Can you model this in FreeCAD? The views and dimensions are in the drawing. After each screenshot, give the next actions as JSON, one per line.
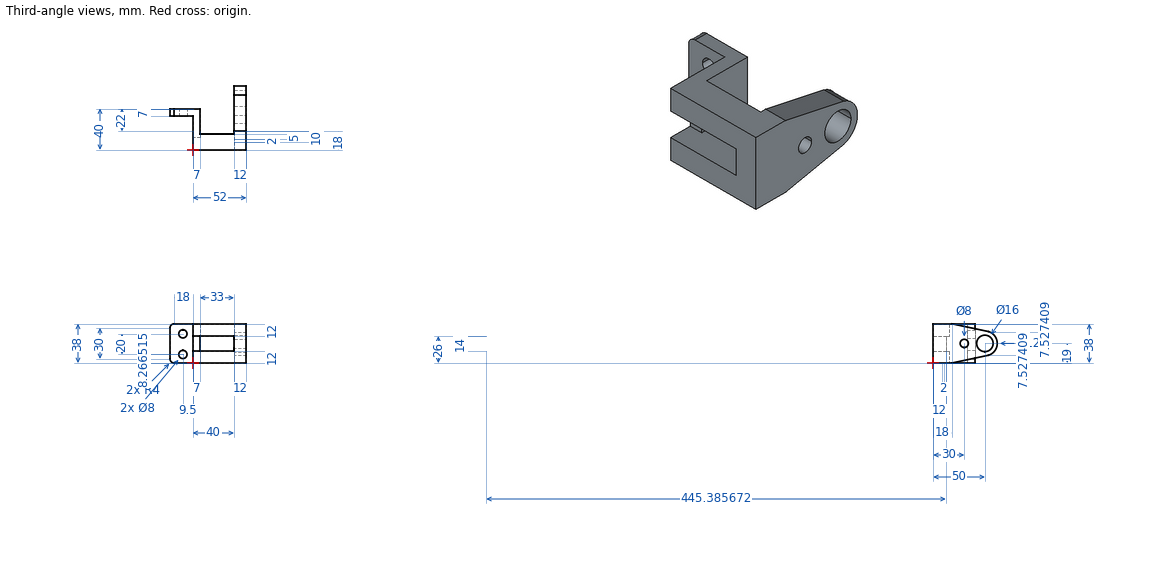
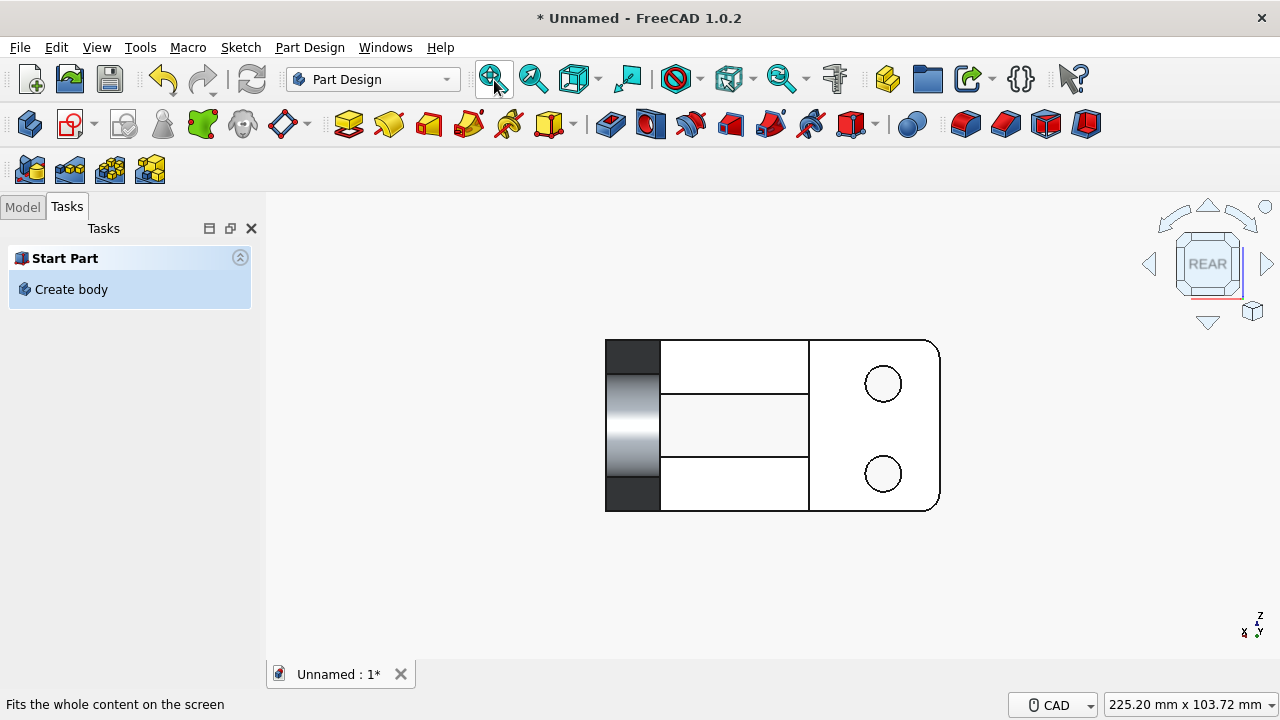
{"action": "left_click", "coordinate": [692, 366]}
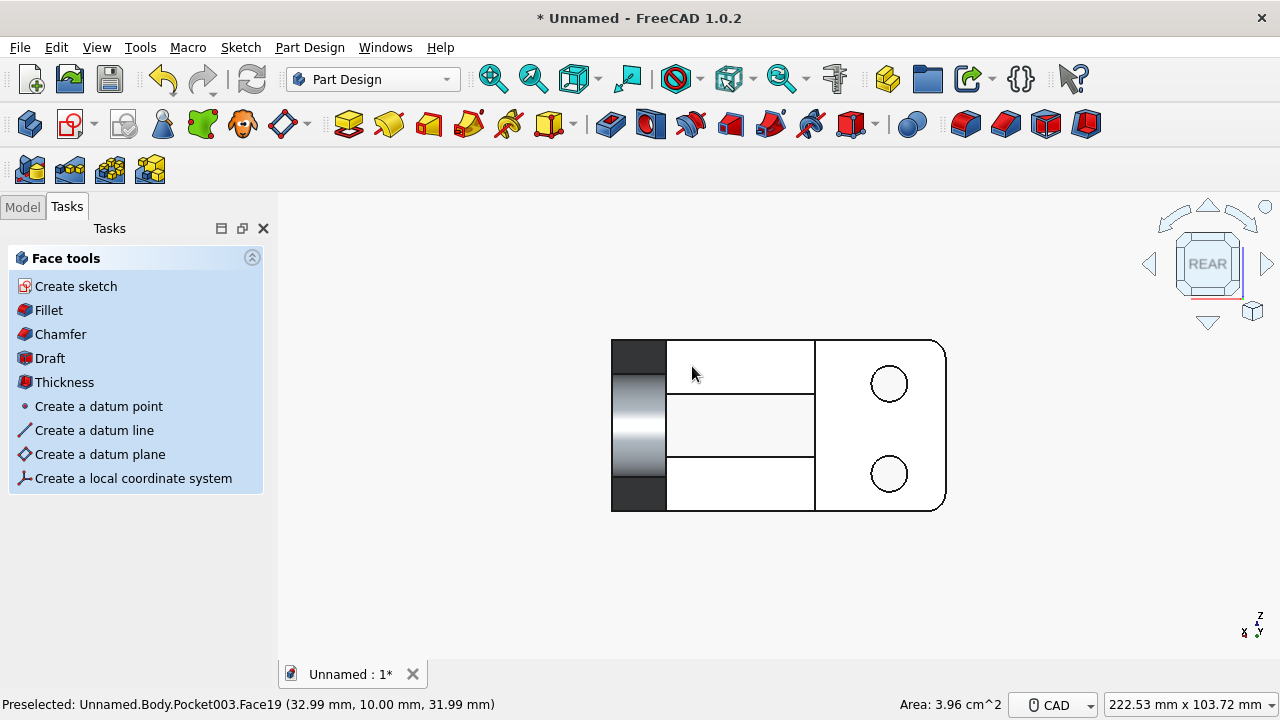
{"action": "left_click", "coordinate": [70, 124]}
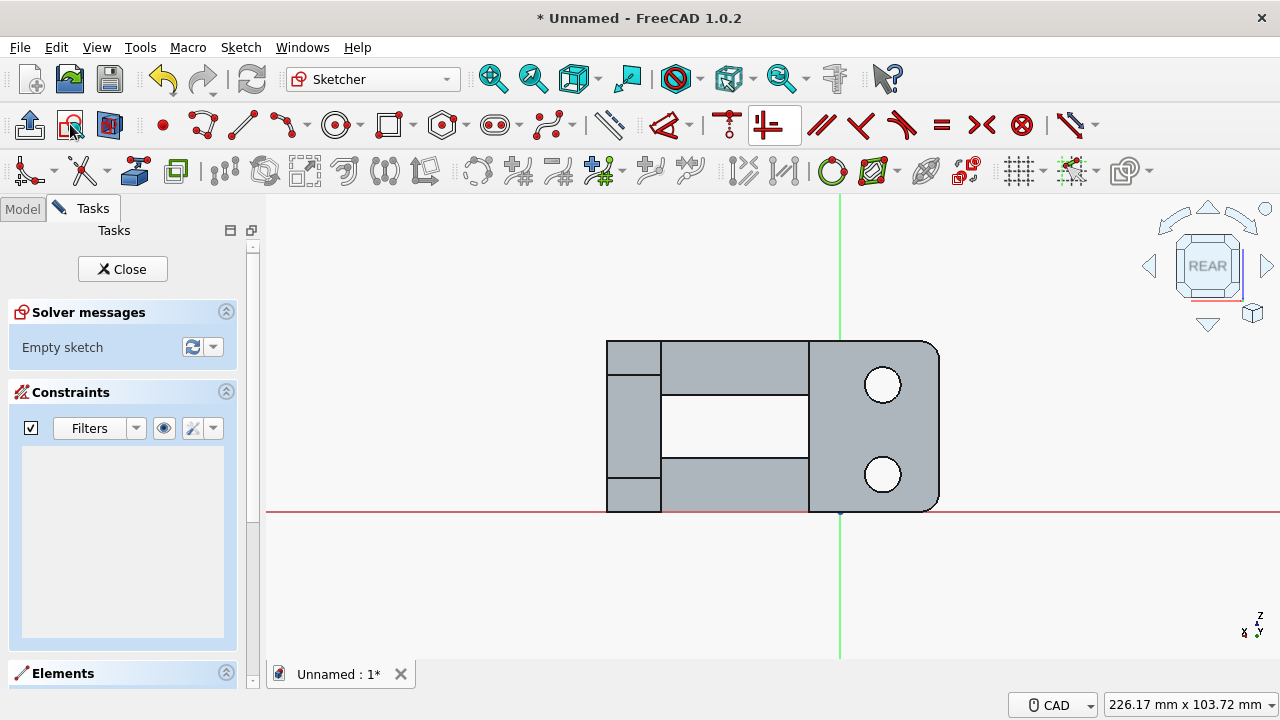
{"action": "scroll", "coordinate": [807, 427], "scroll_direction": "up", "scroll_amount": 3}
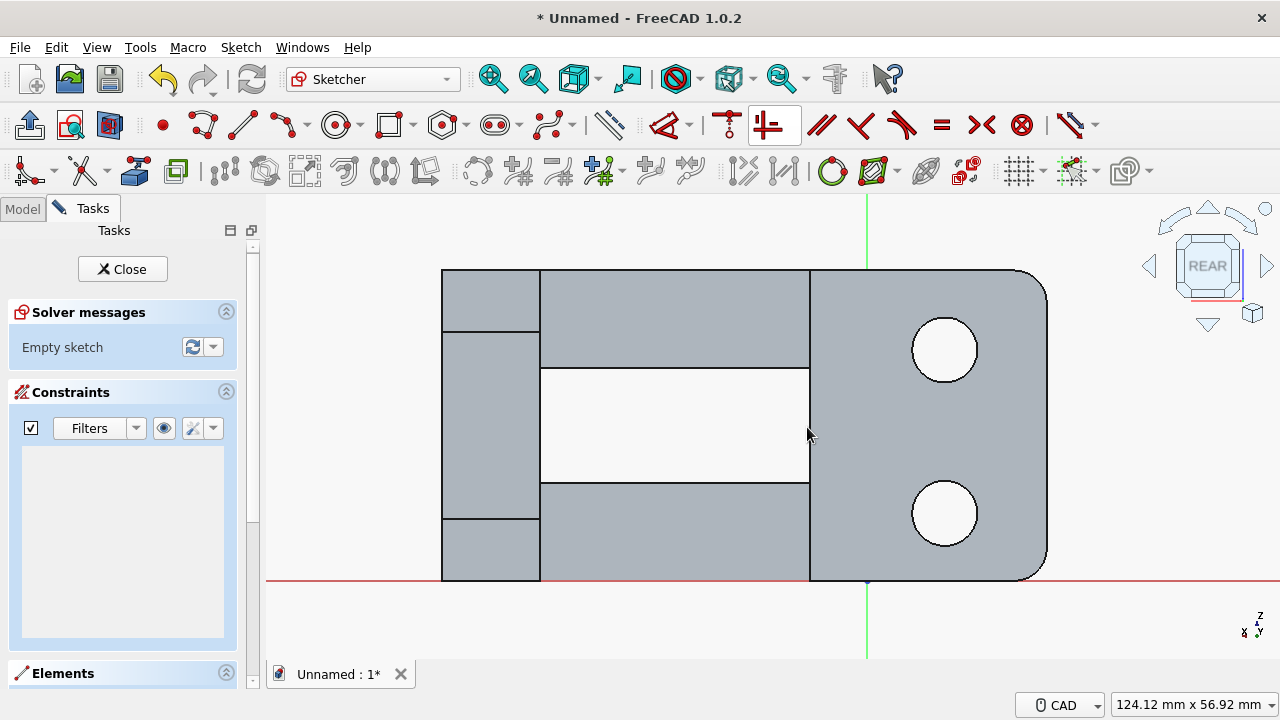
{"action": "left_click", "coordinate": [390, 126]}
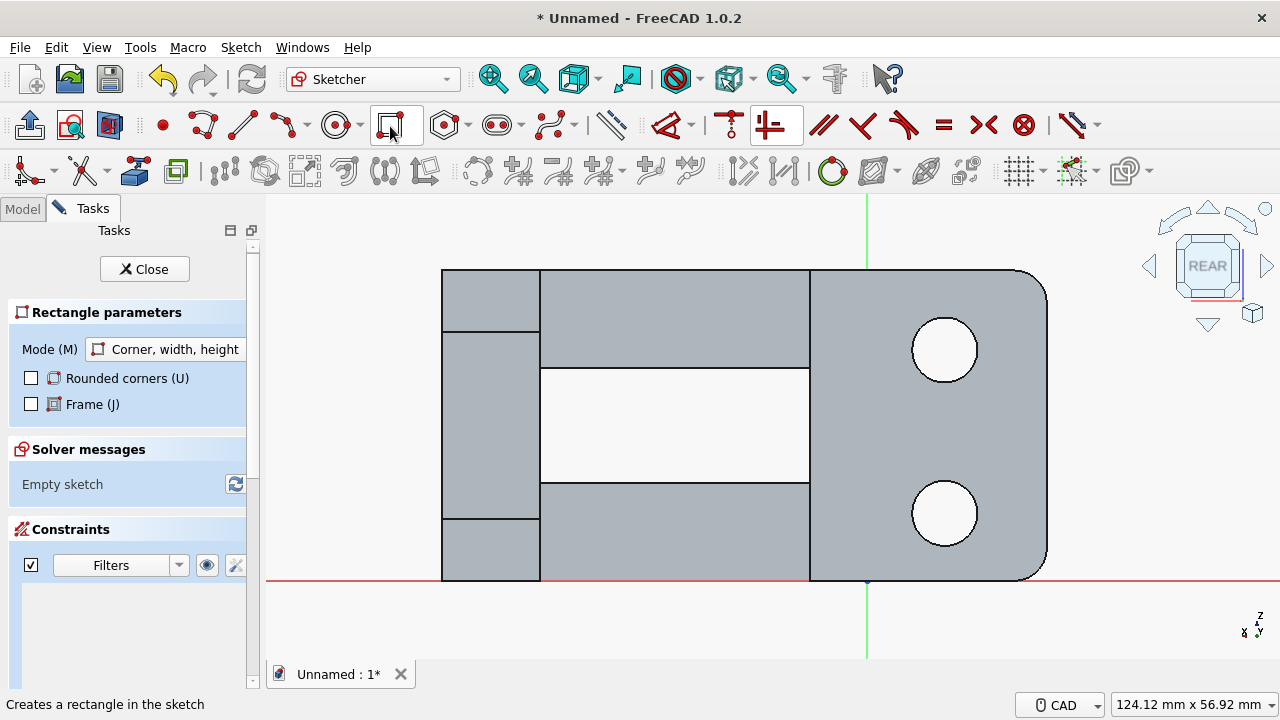
{"action": "left_click", "coordinate": [540, 270]}
{"action": "left_click", "coordinate": [810, 368]}
{"action": "key", "text": "Escape"}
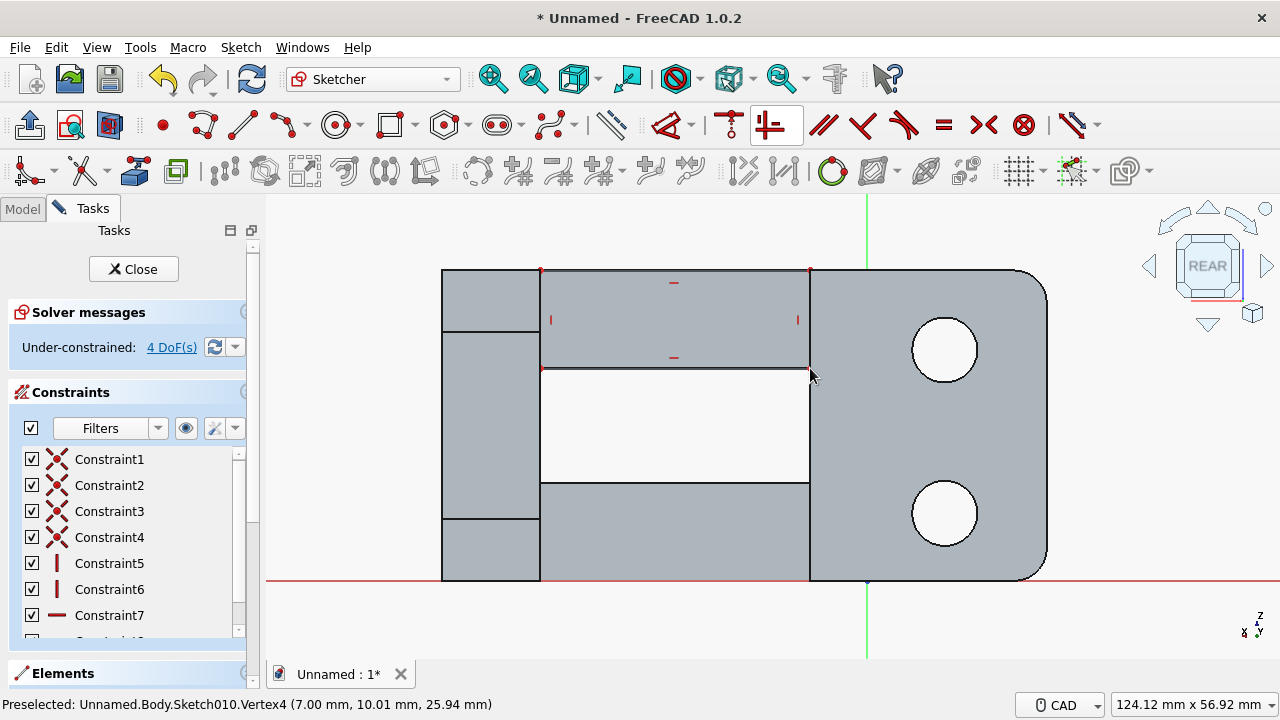
{"action": "left_click", "coordinate": [666, 126]}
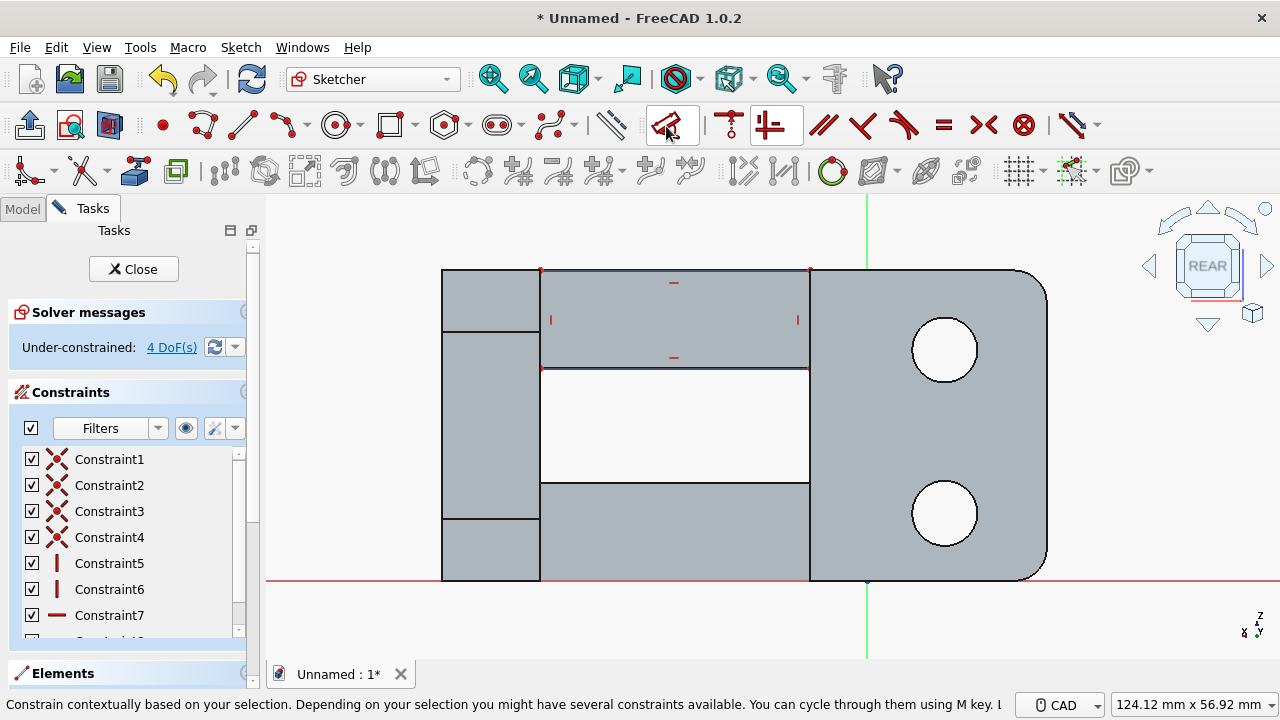
{"action": "left_click", "coordinate": [540, 300]}
{"action": "left_click", "coordinate": [506, 320]}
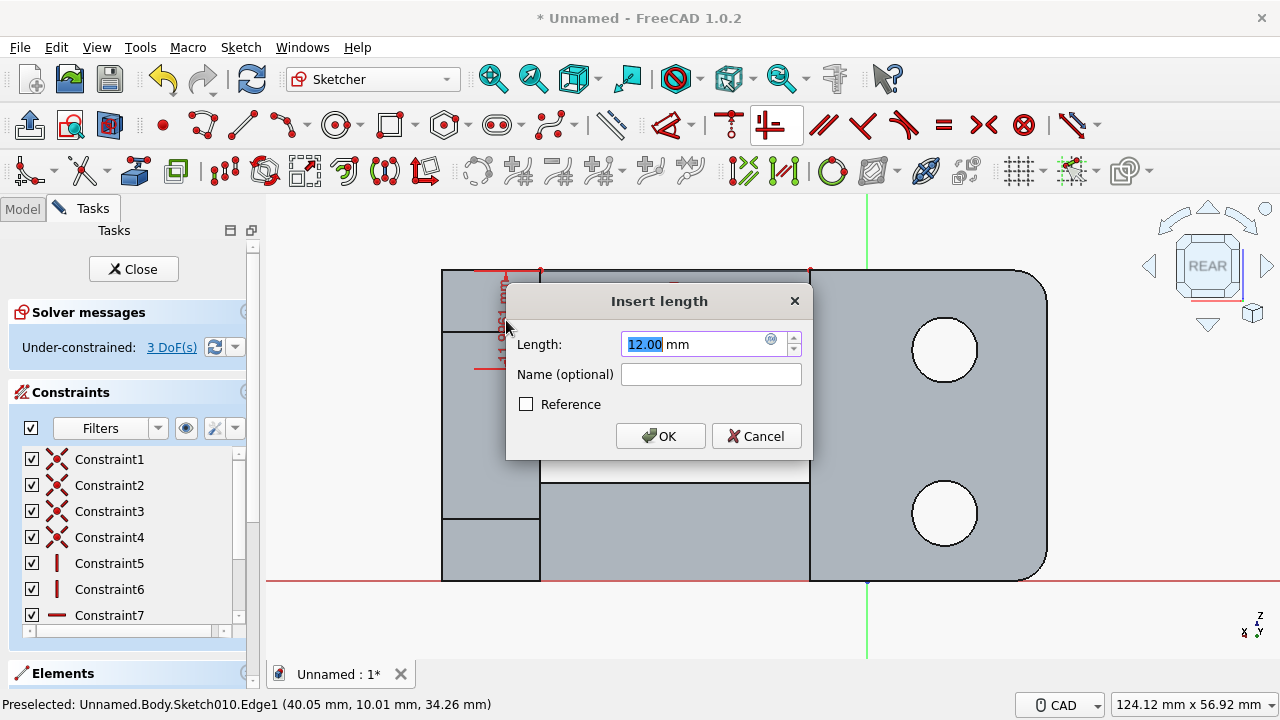
{"action": "type", "text": "12"}
{"action": "key", "text": "Return"}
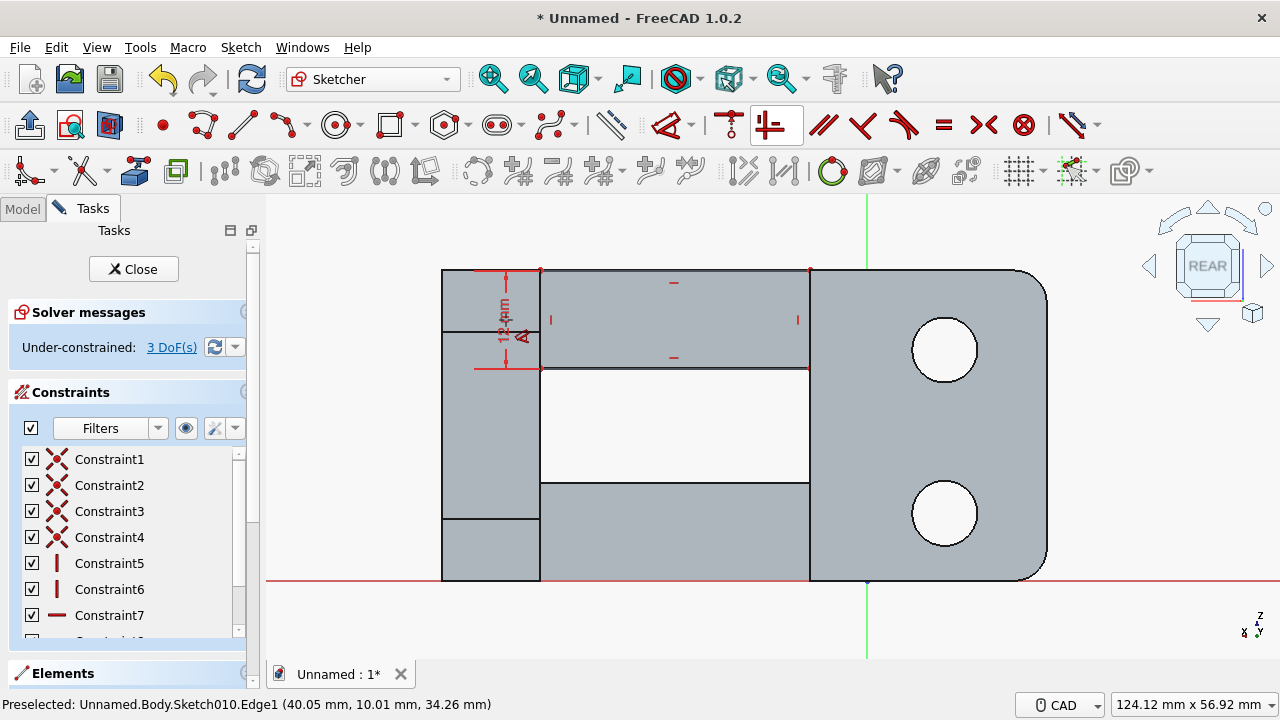
{"action": "left_click", "coordinate": [621, 369]}
{"action": "left_click", "coordinate": [675, 335]}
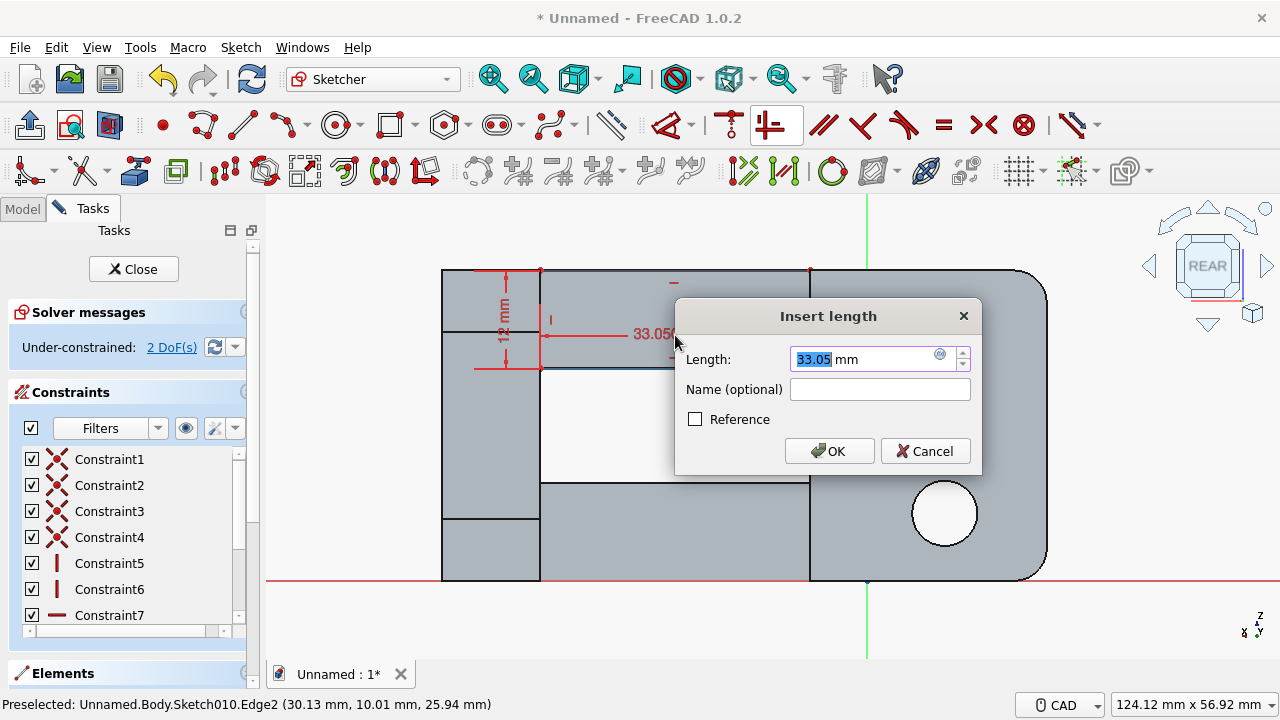
{"action": "type", "text": "33"}
{"action": "key", "text": "Return"}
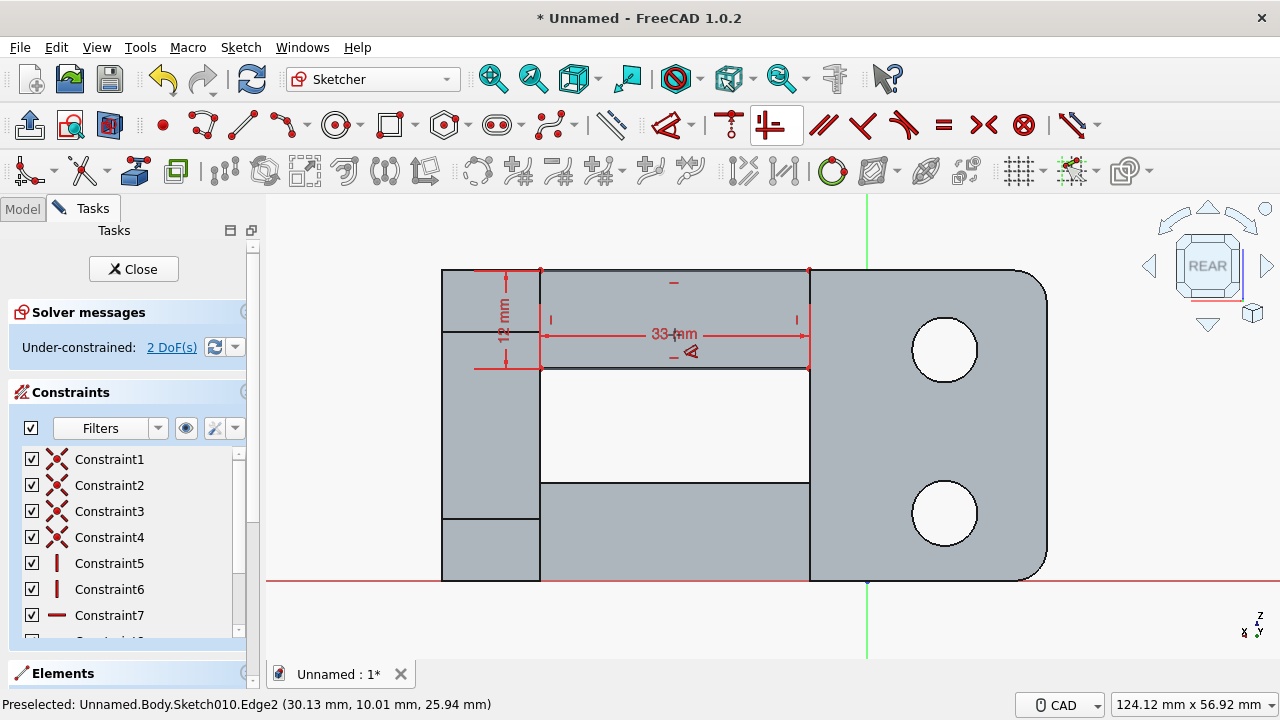
{"action": "left_click", "coordinate": [810, 369]}
{"action": "left_click", "coordinate": [838, 615]}